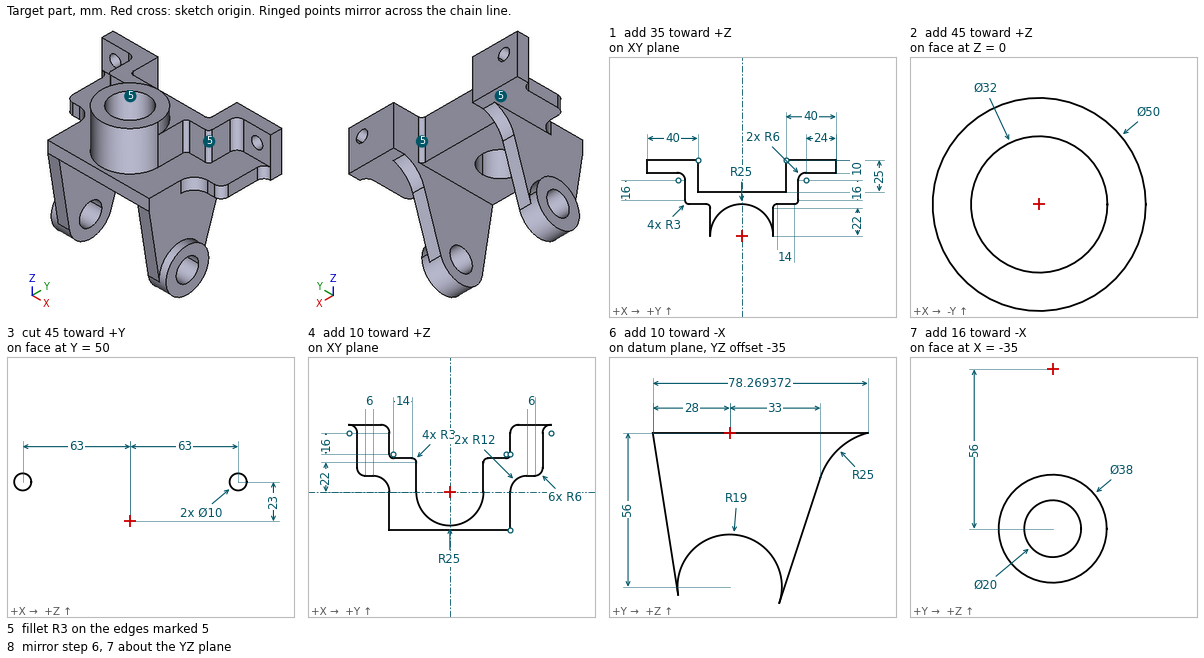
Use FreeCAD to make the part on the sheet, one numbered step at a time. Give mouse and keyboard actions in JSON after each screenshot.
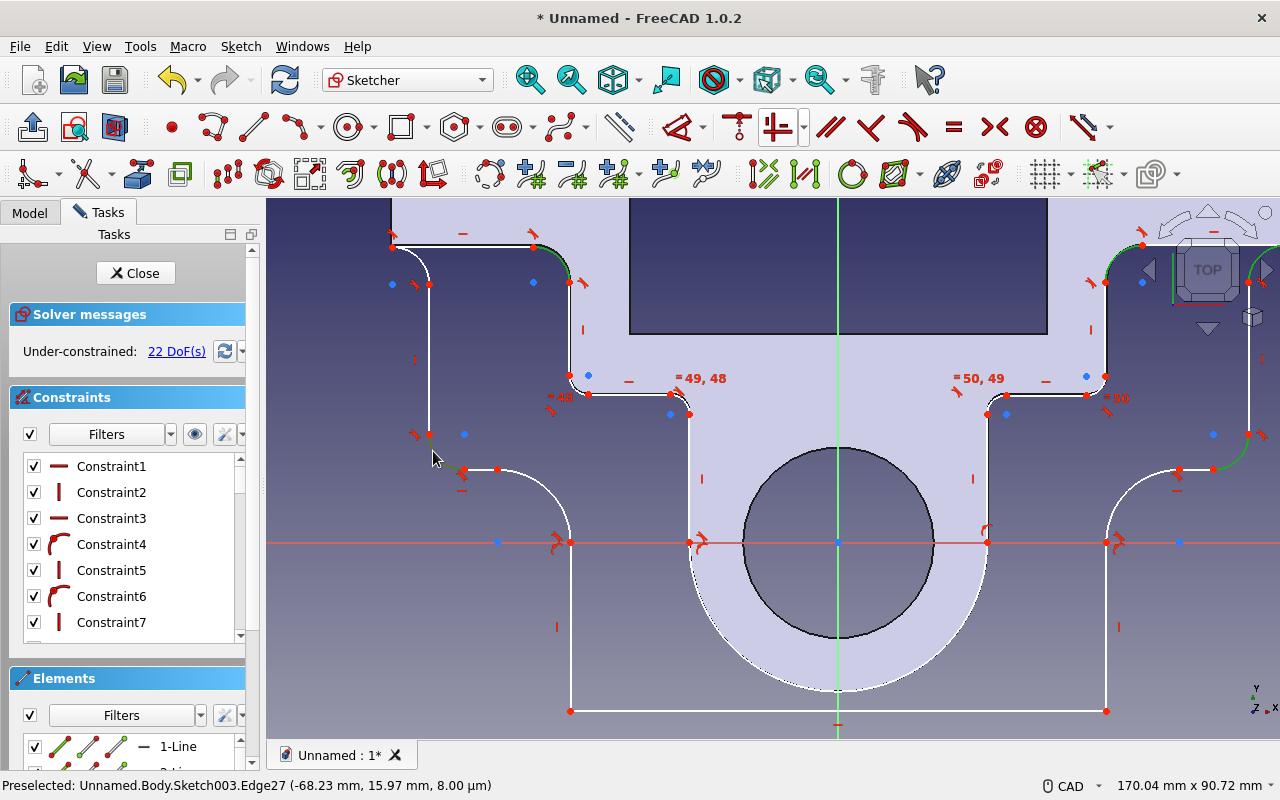
{"action": "left_click", "coordinate": [425, 267]}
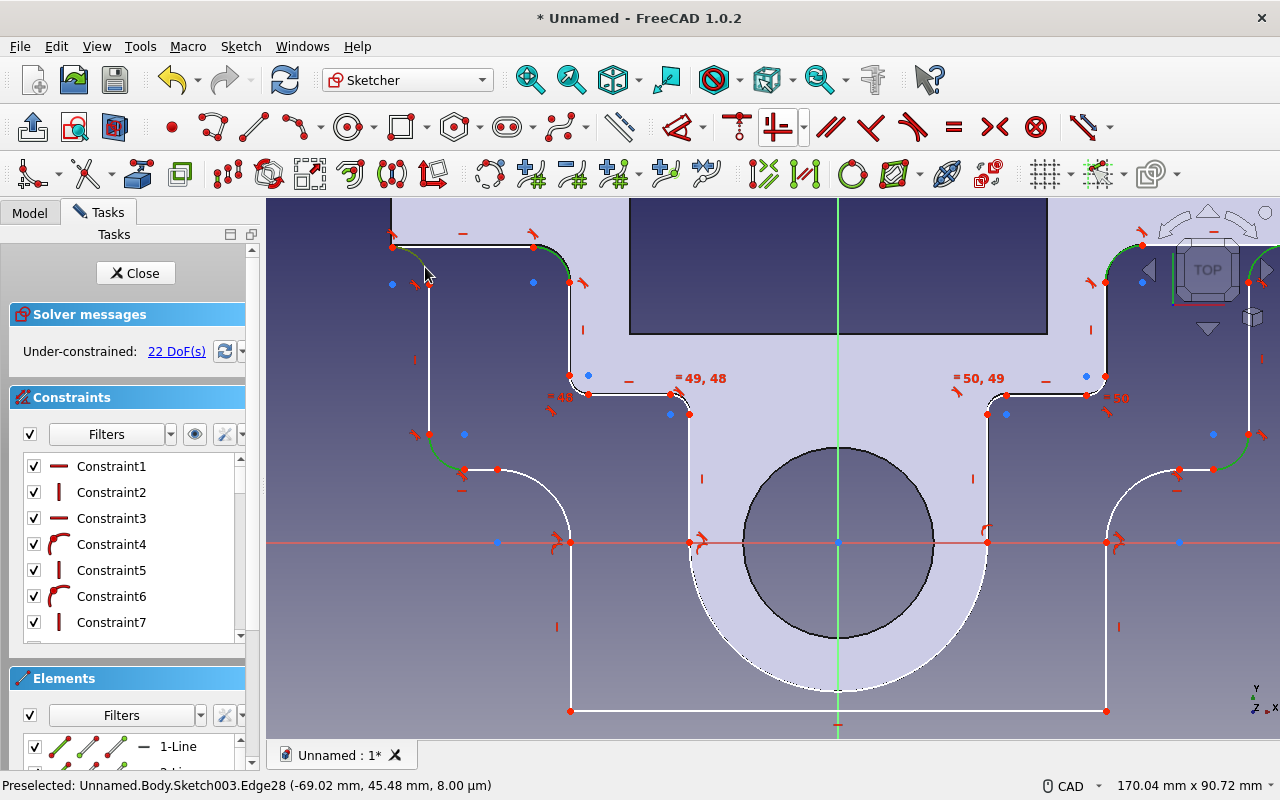
{"action": "left_click", "coordinate": [954, 128]}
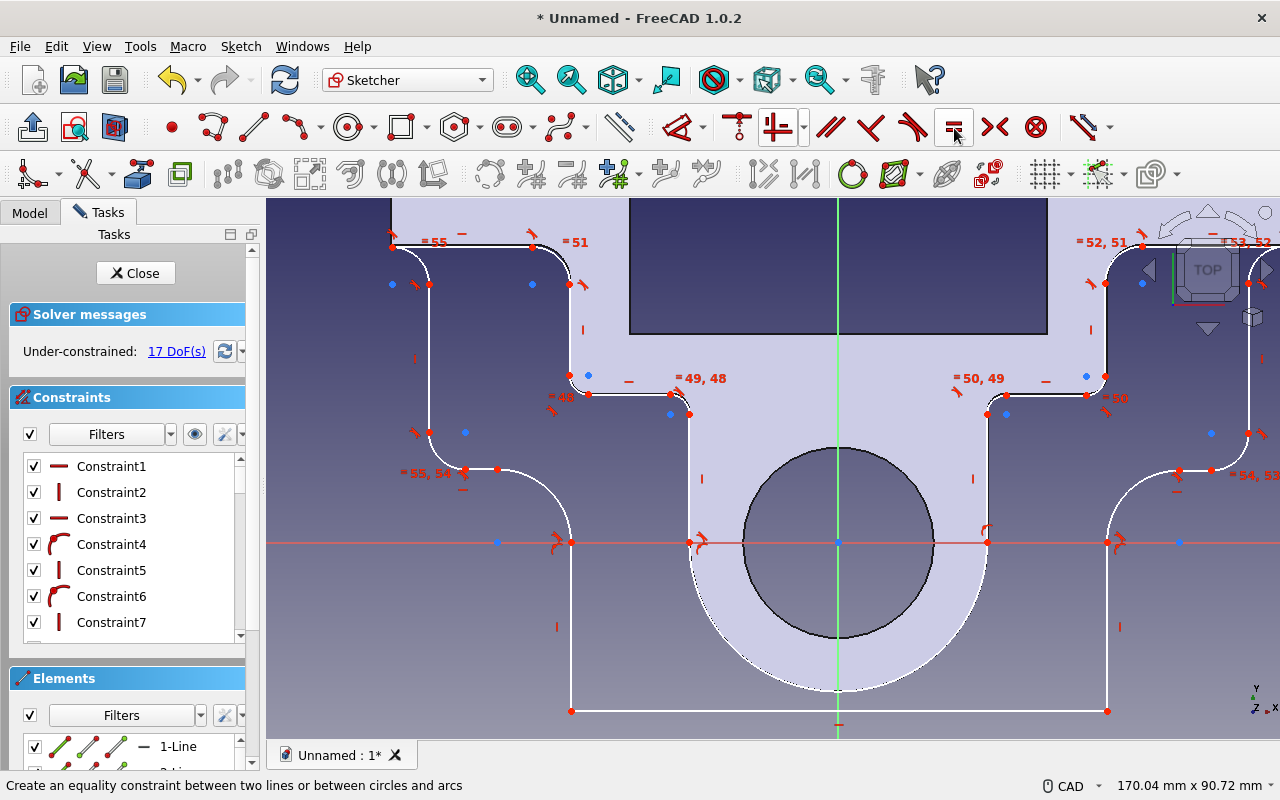
{"action": "left_click", "coordinate": [1115, 510]}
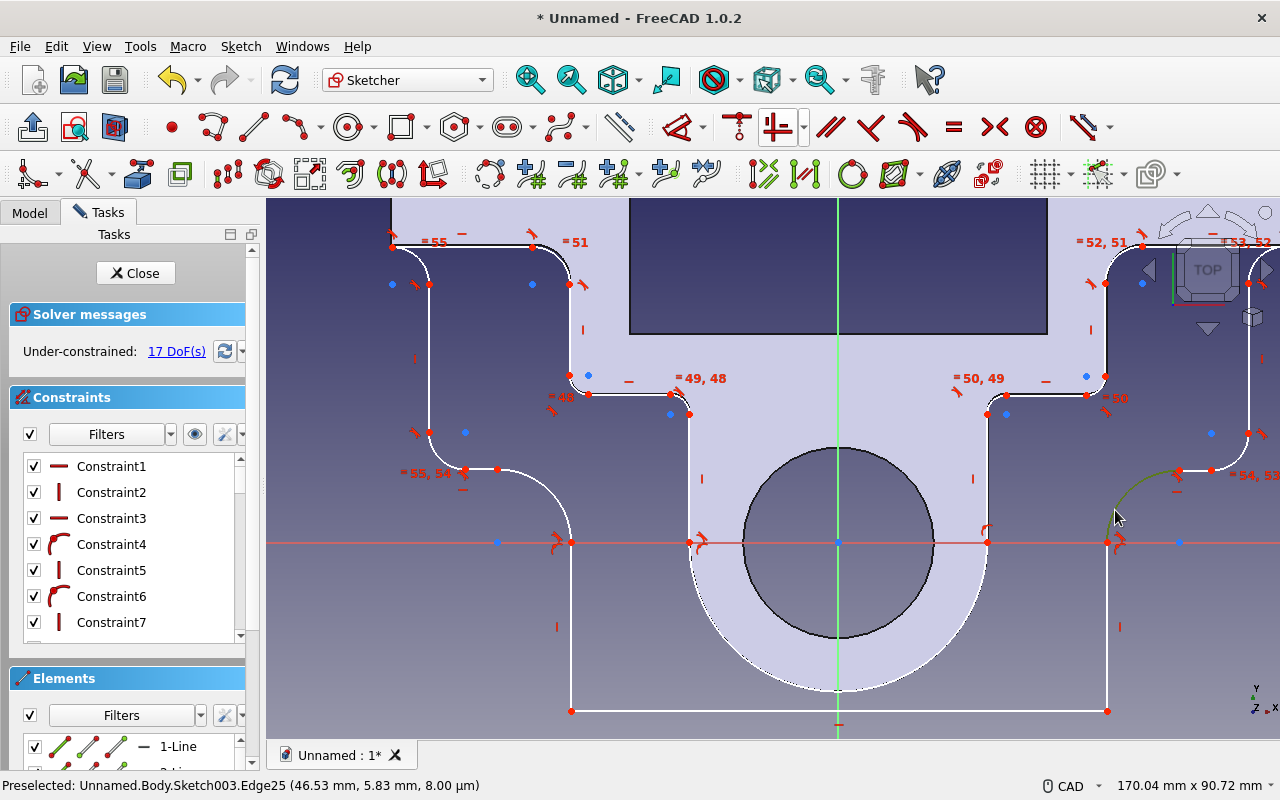
{"action": "left_click", "coordinate": [563, 509]}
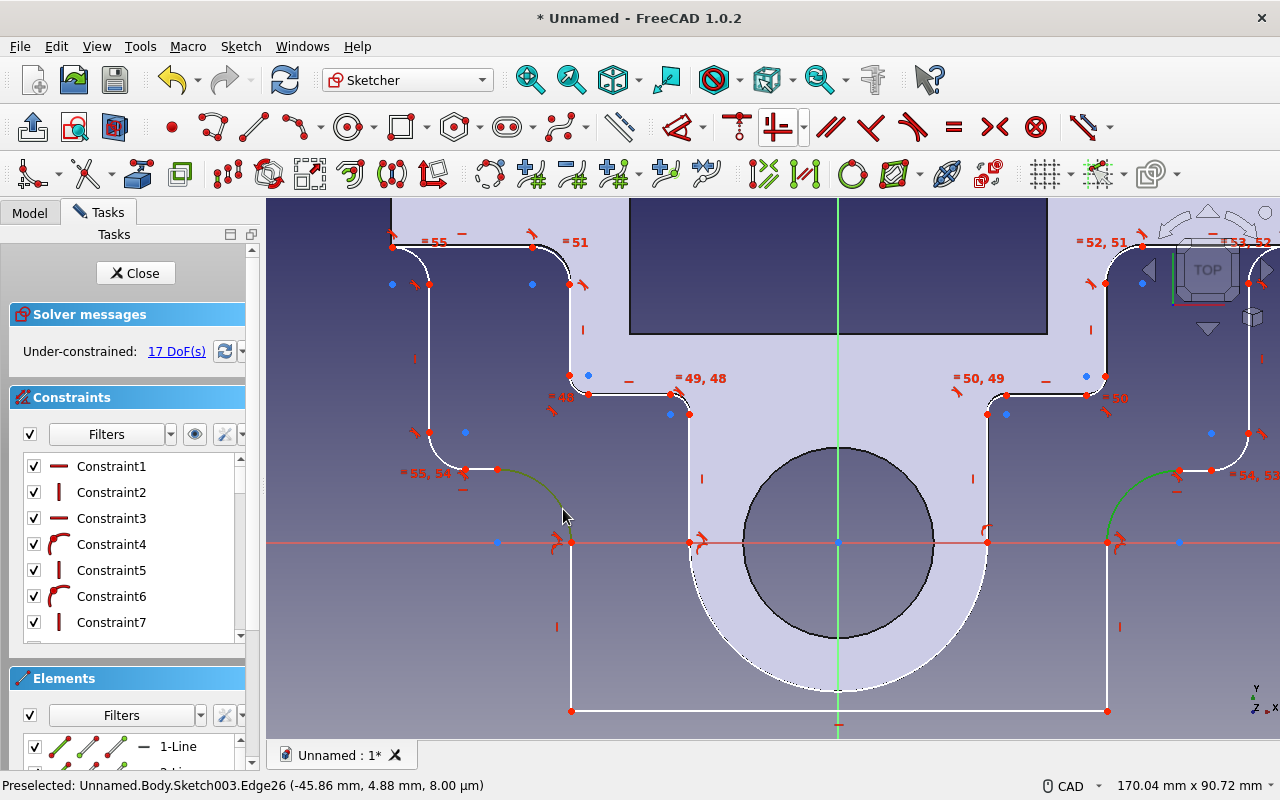
{"action": "left_click", "coordinate": [954, 128]}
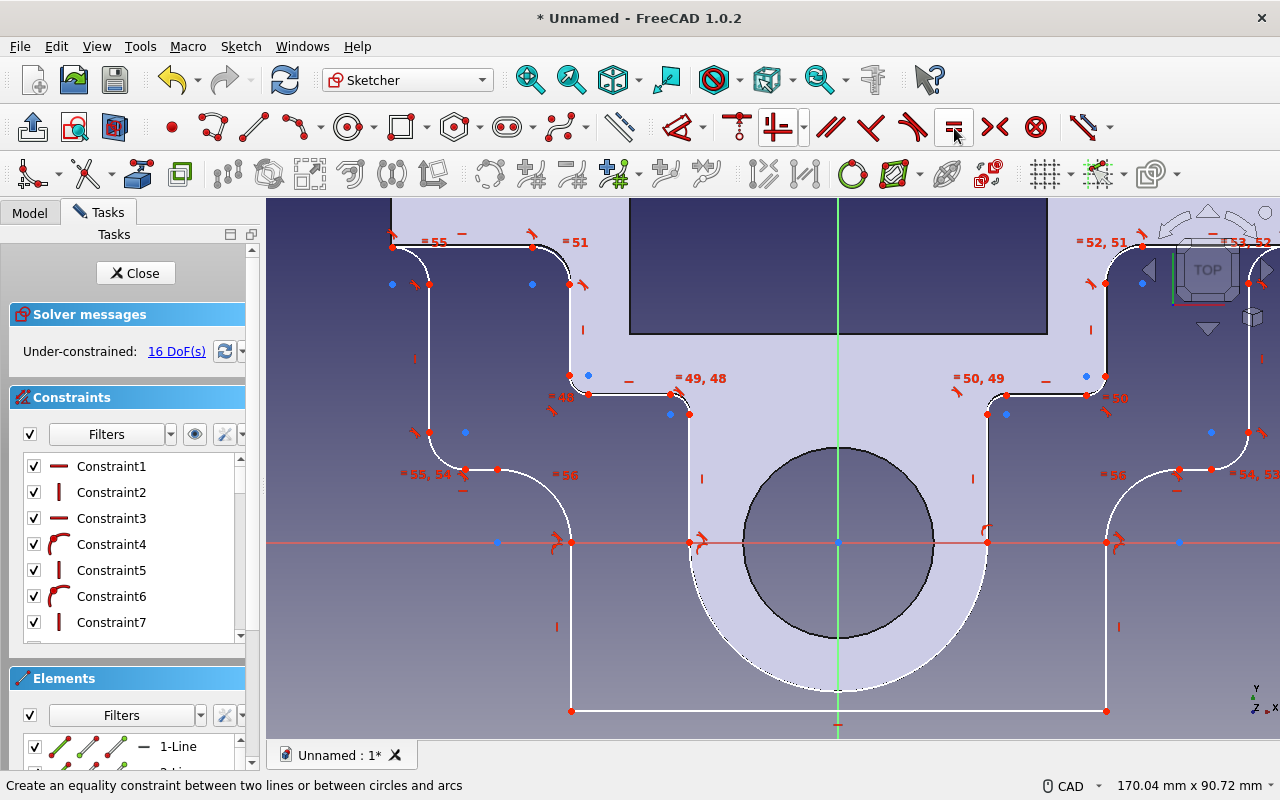
{"action": "left_click", "coordinate": [838, 543]}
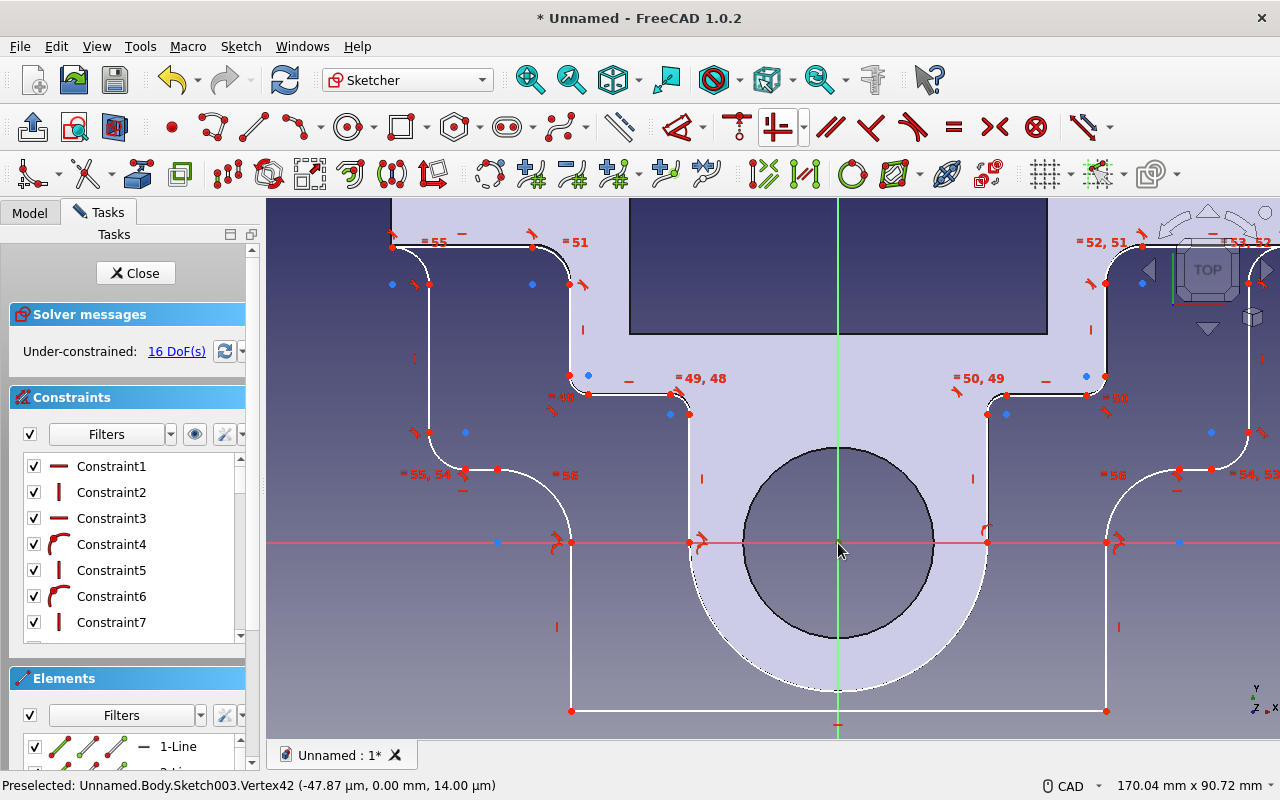
{"action": "left_click", "coordinate": [838, 642]}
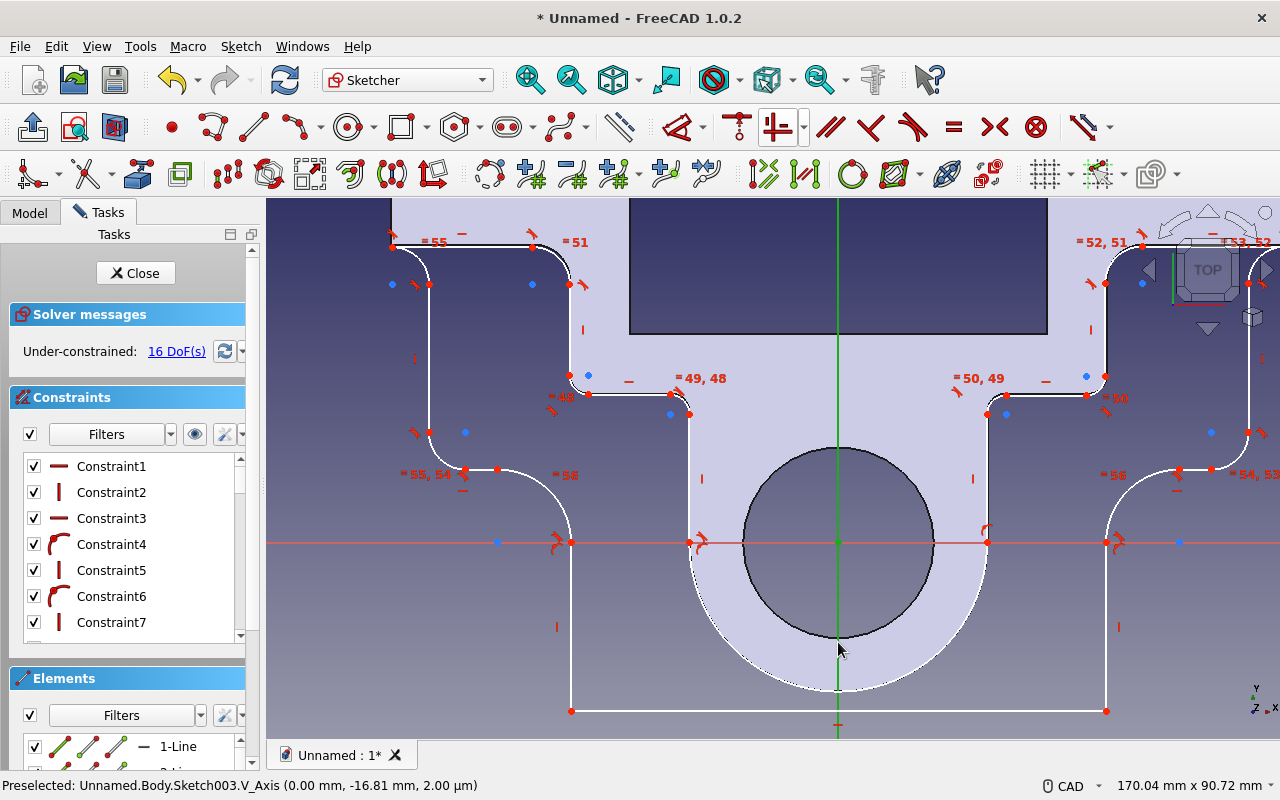
{"action": "left_click", "coordinate": [737, 128]}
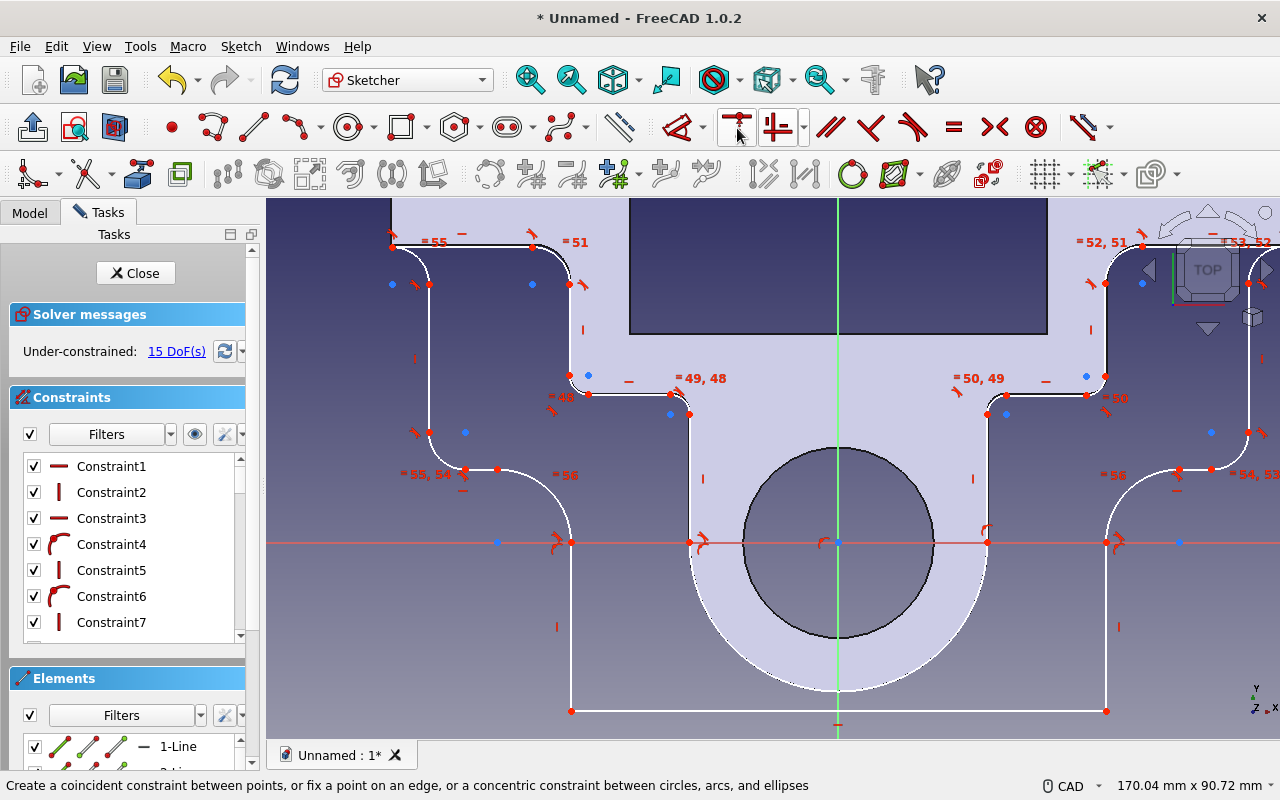
{"action": "left_click", "coordinate": [589, 376]}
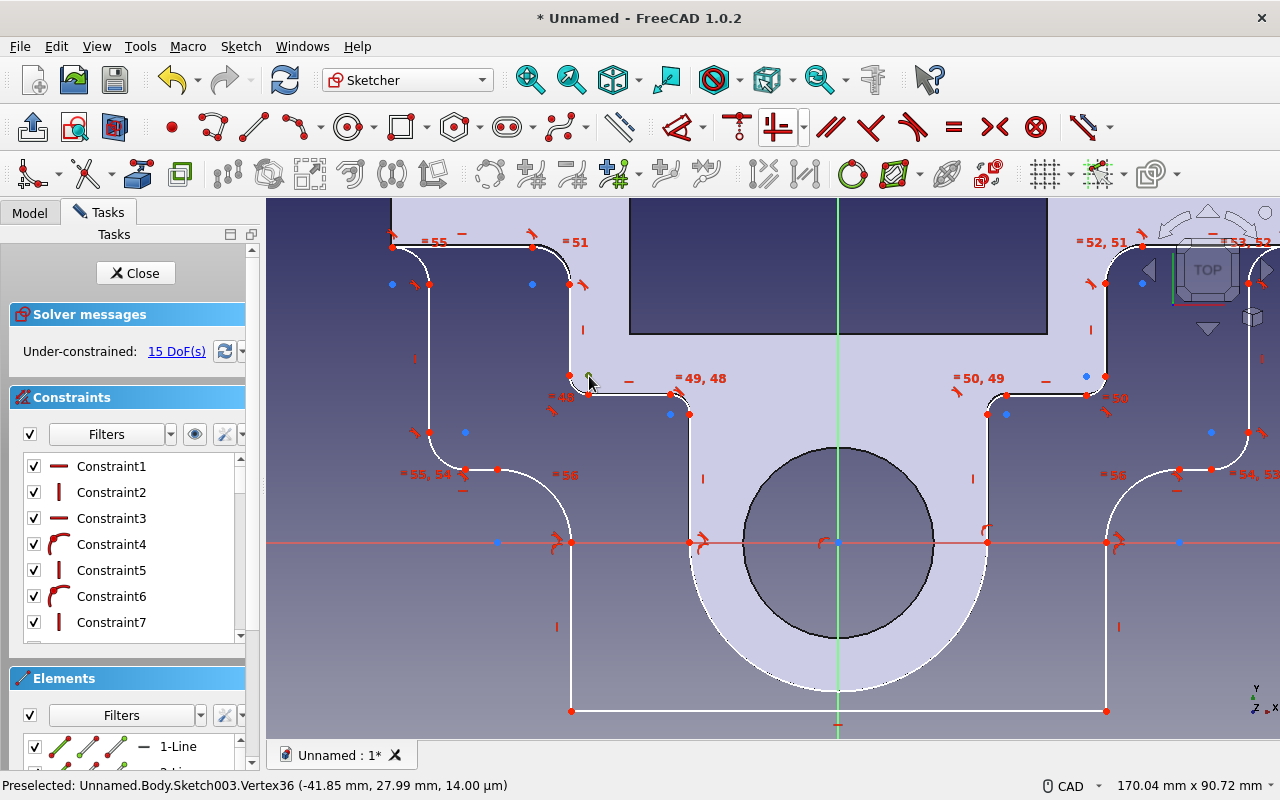
{"action": "left_click", "coordinate": [1086, 376]}